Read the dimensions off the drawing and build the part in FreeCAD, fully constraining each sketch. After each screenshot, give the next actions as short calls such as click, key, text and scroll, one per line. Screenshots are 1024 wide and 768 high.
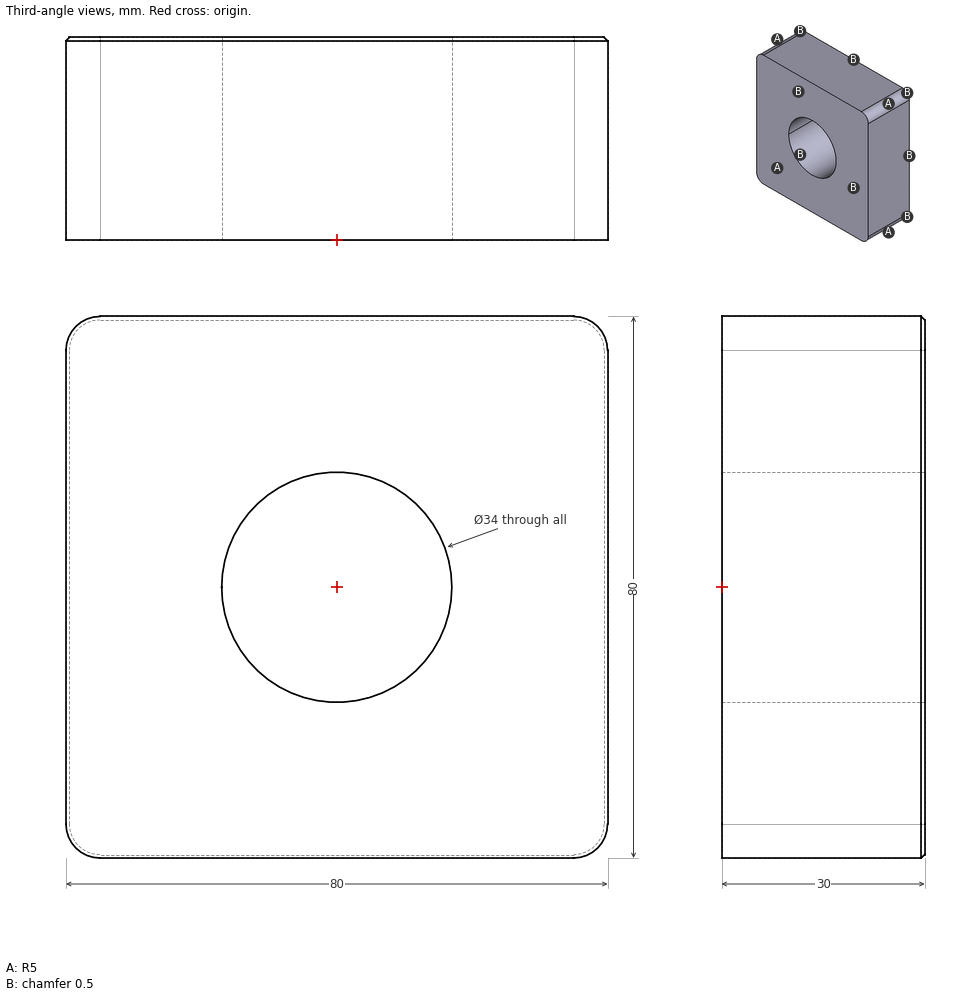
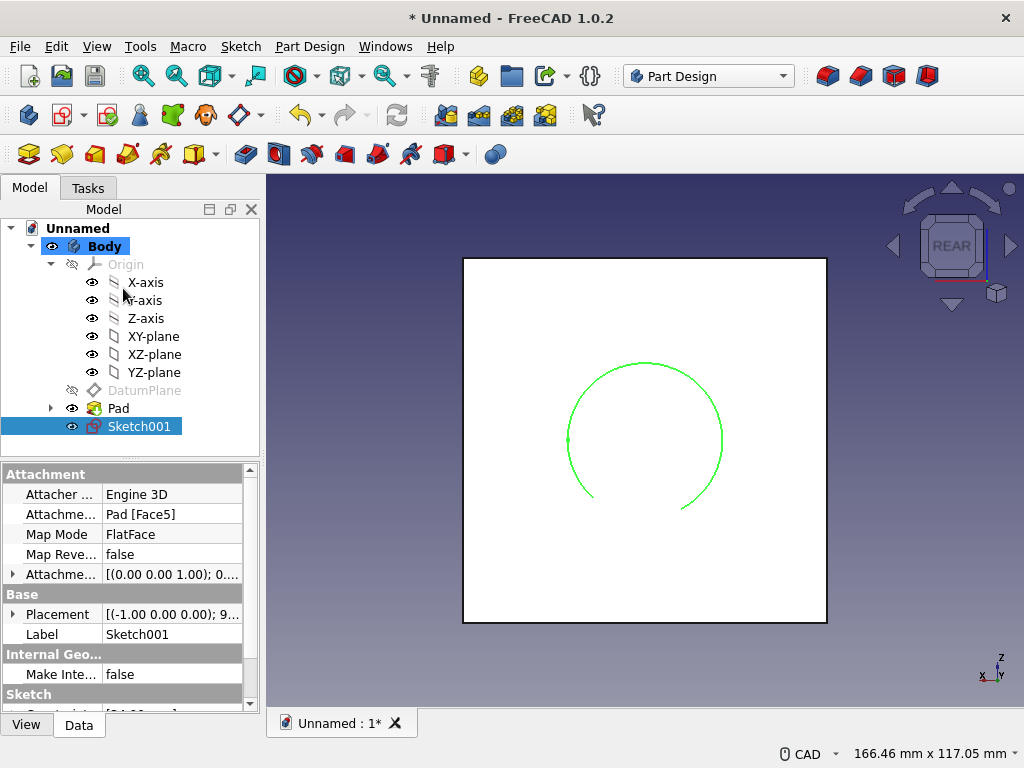
click(279, 154)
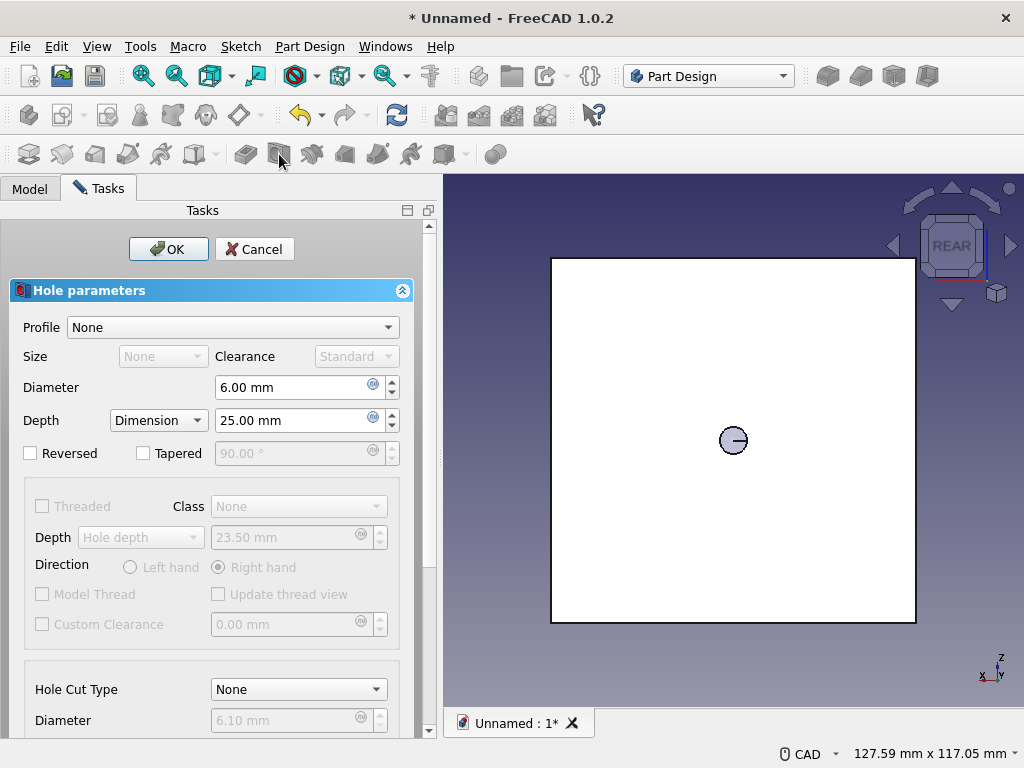
triple_click(300, 388)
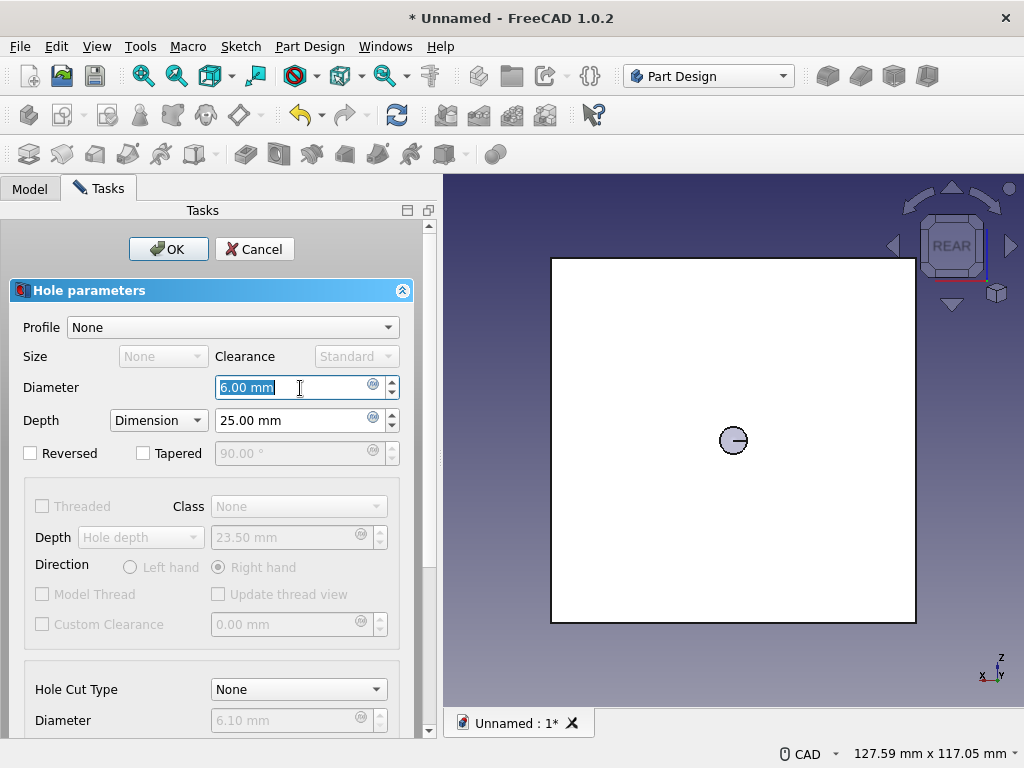
text(34)
key(Tab)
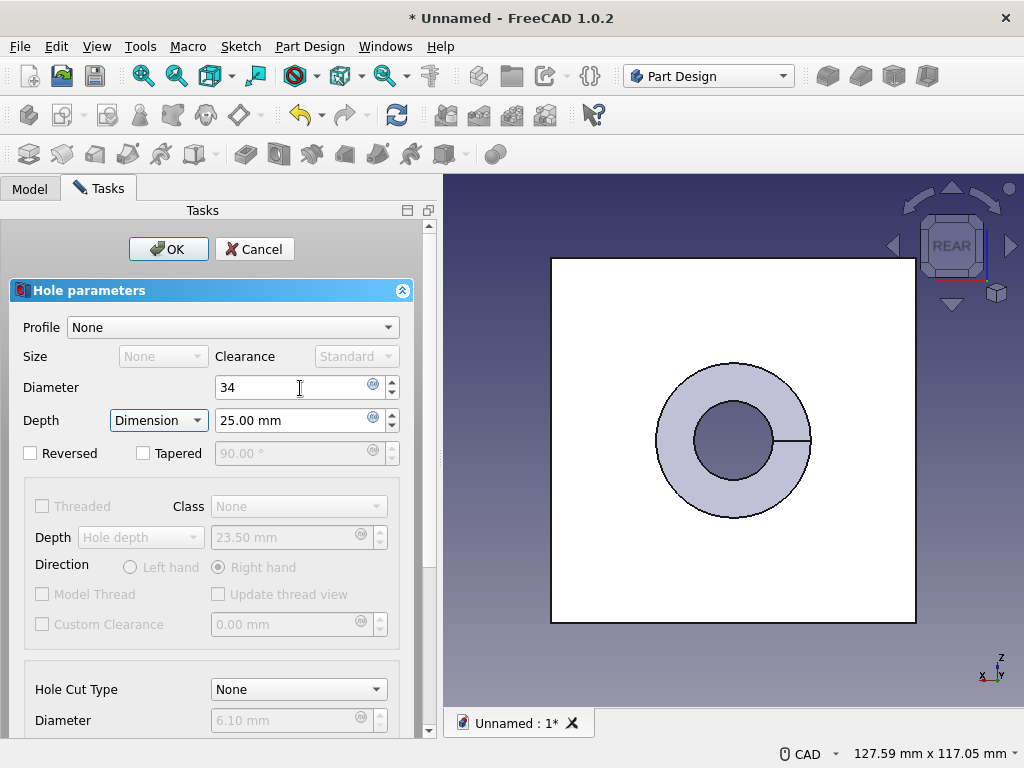
click(160, 420)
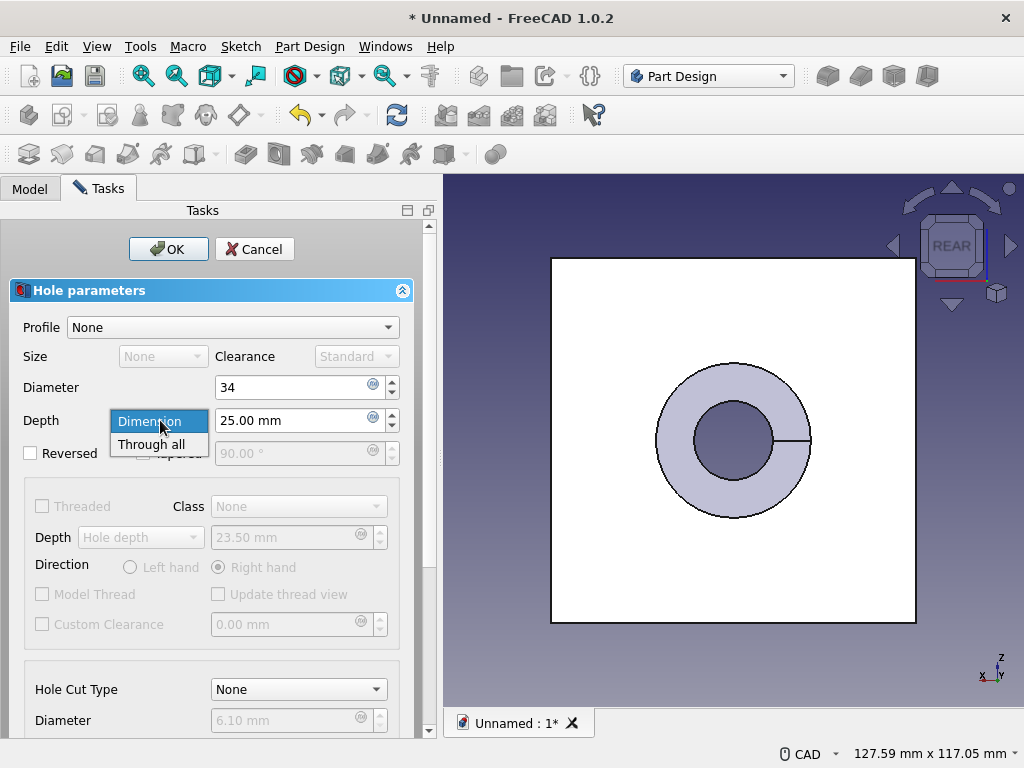
click(158, 444)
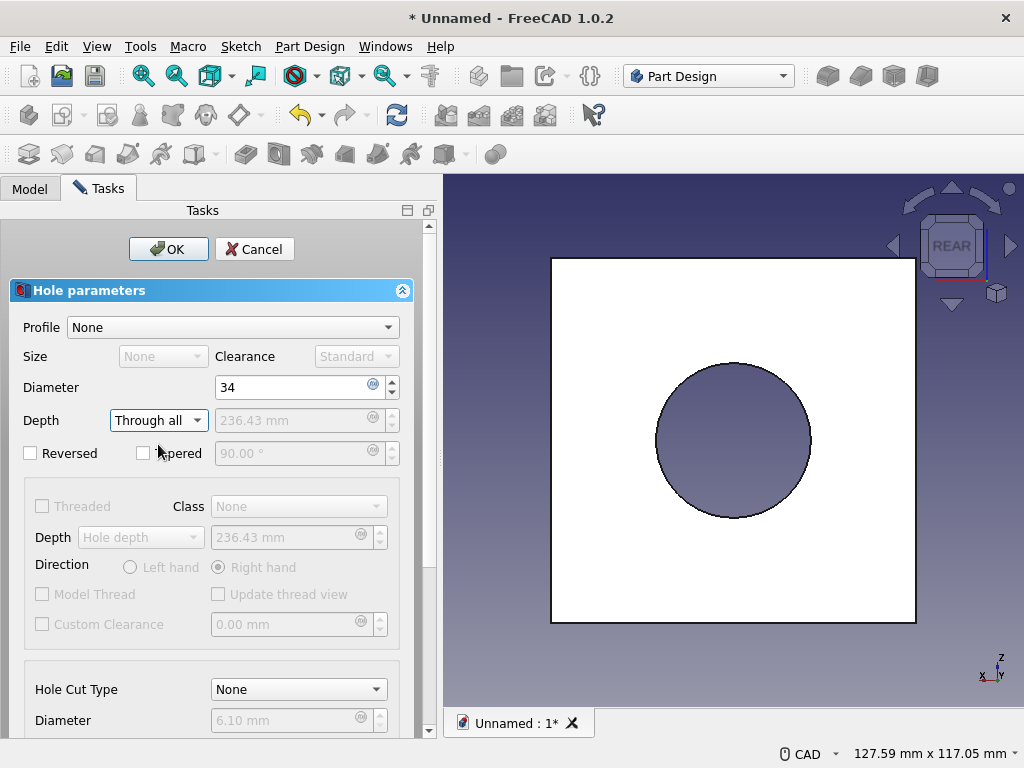
click(169, 249)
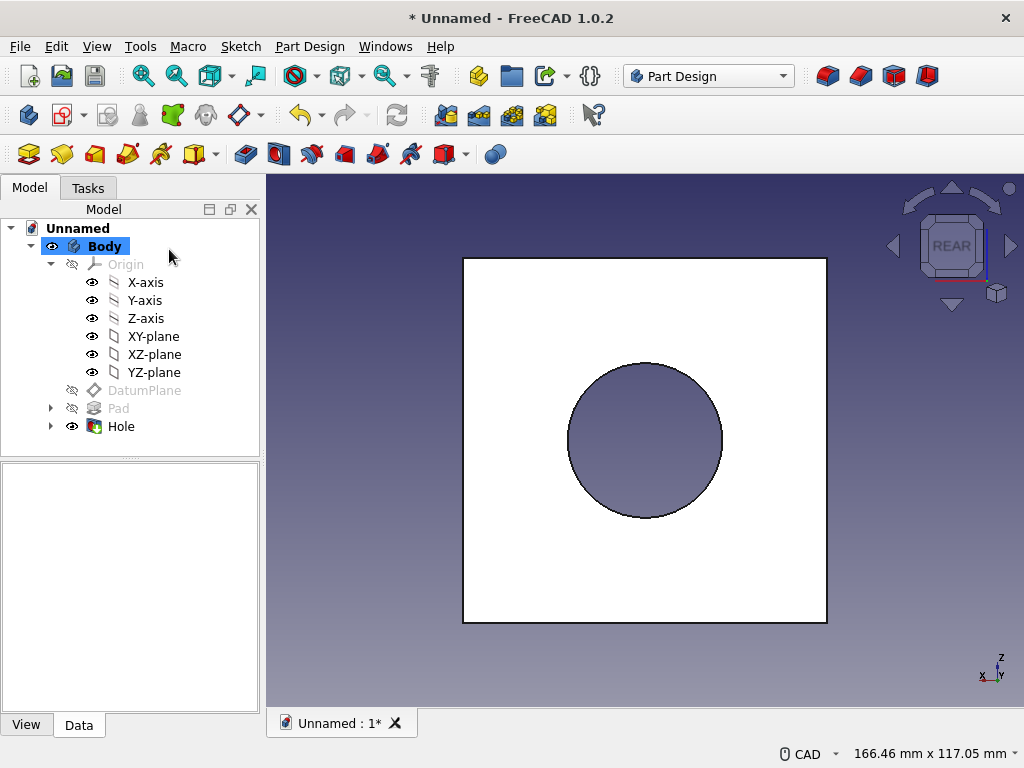
key(0)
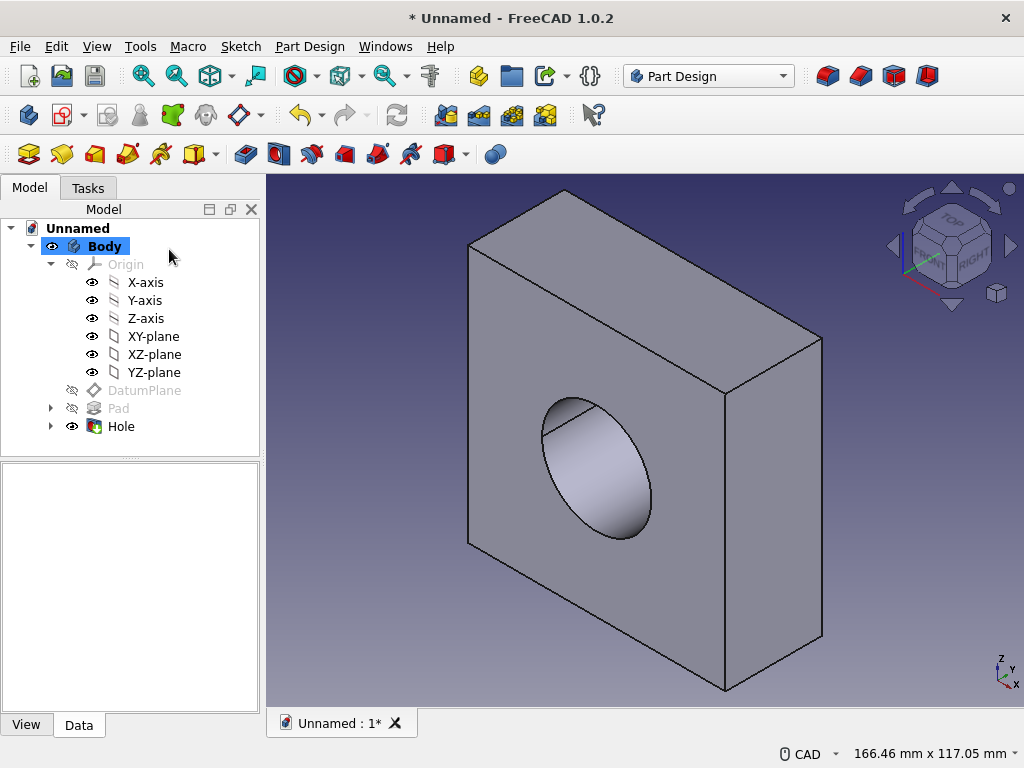
click(774, 365)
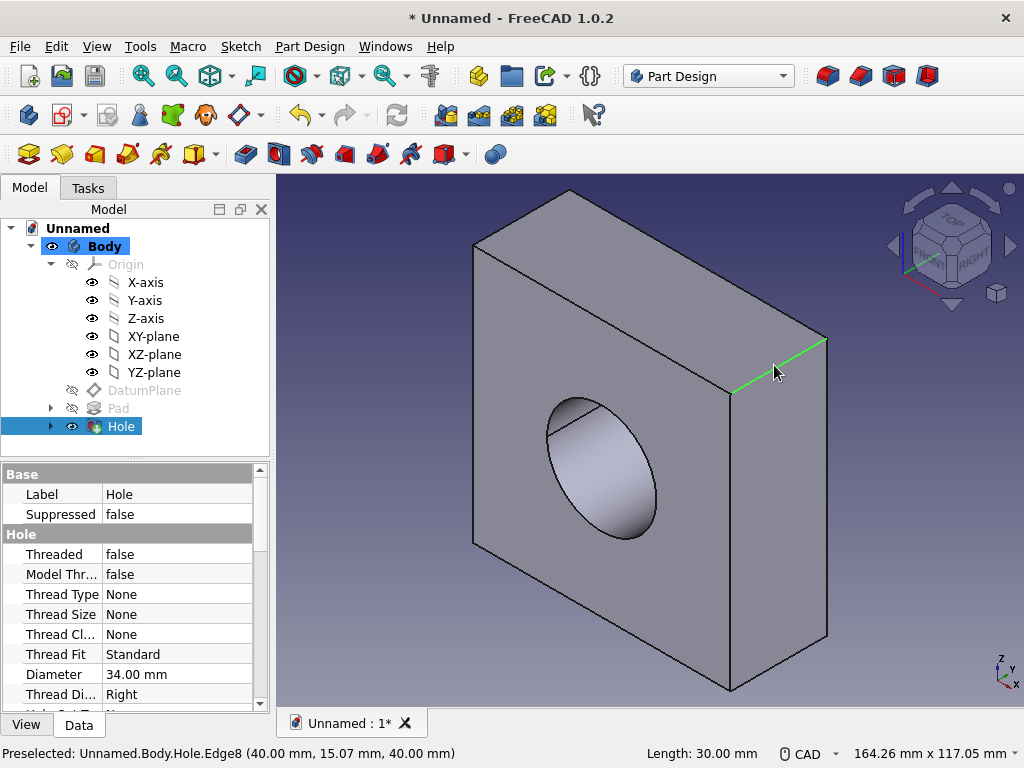
key(2)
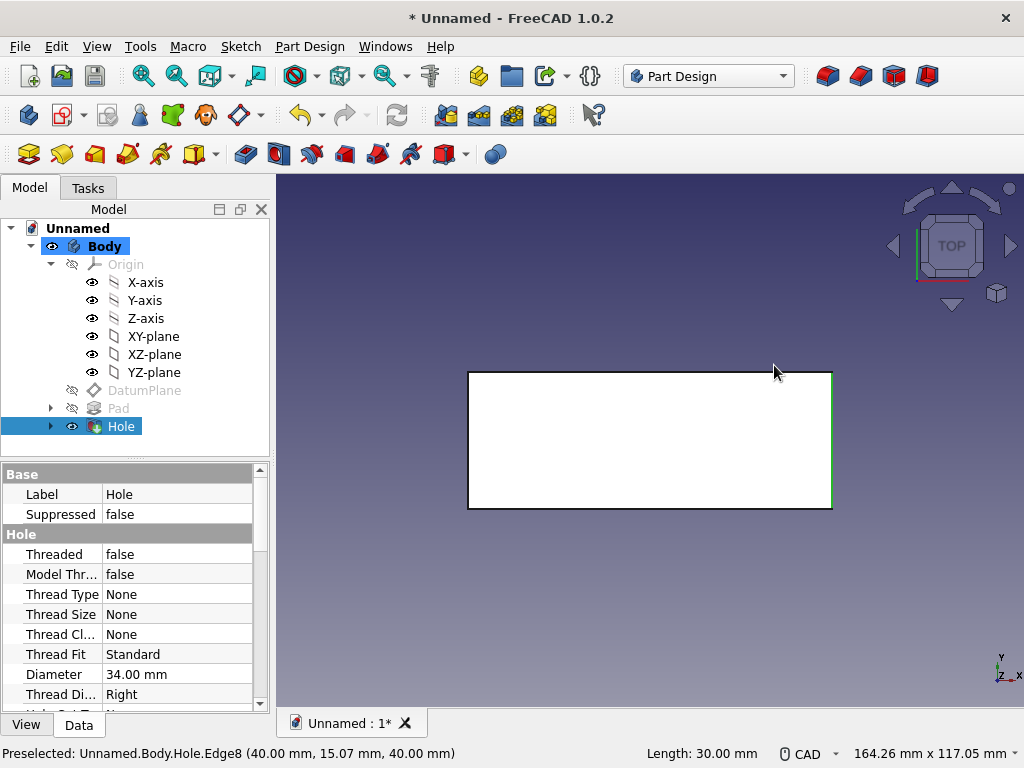
click(468, 439, ctrl)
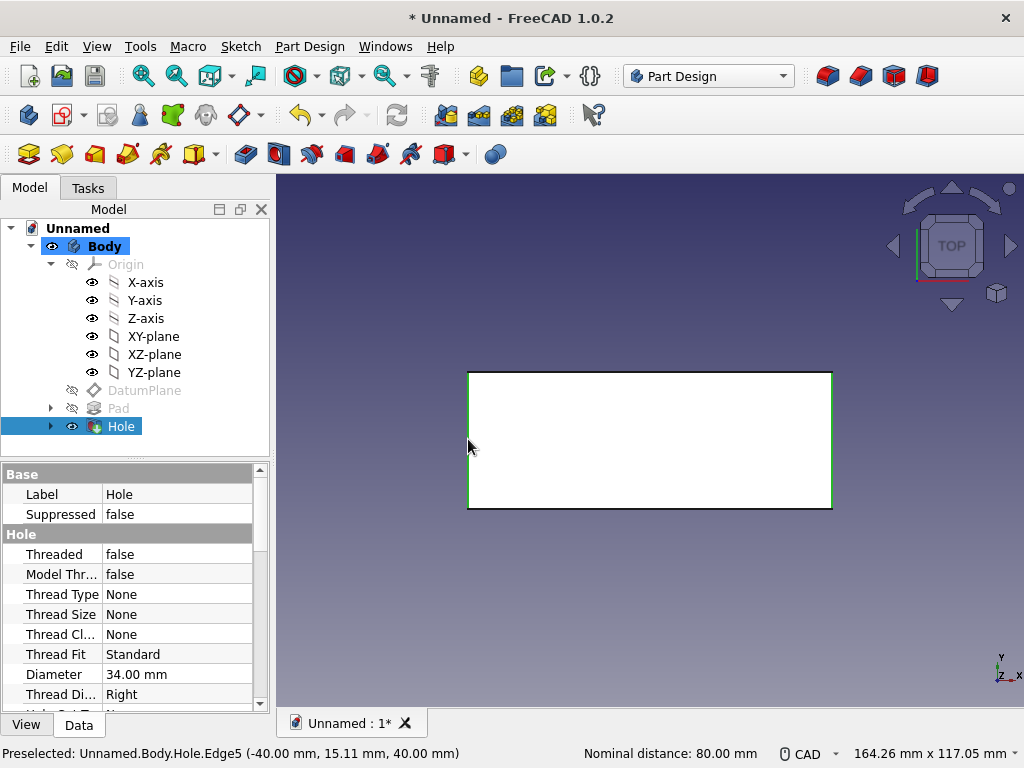
key(1)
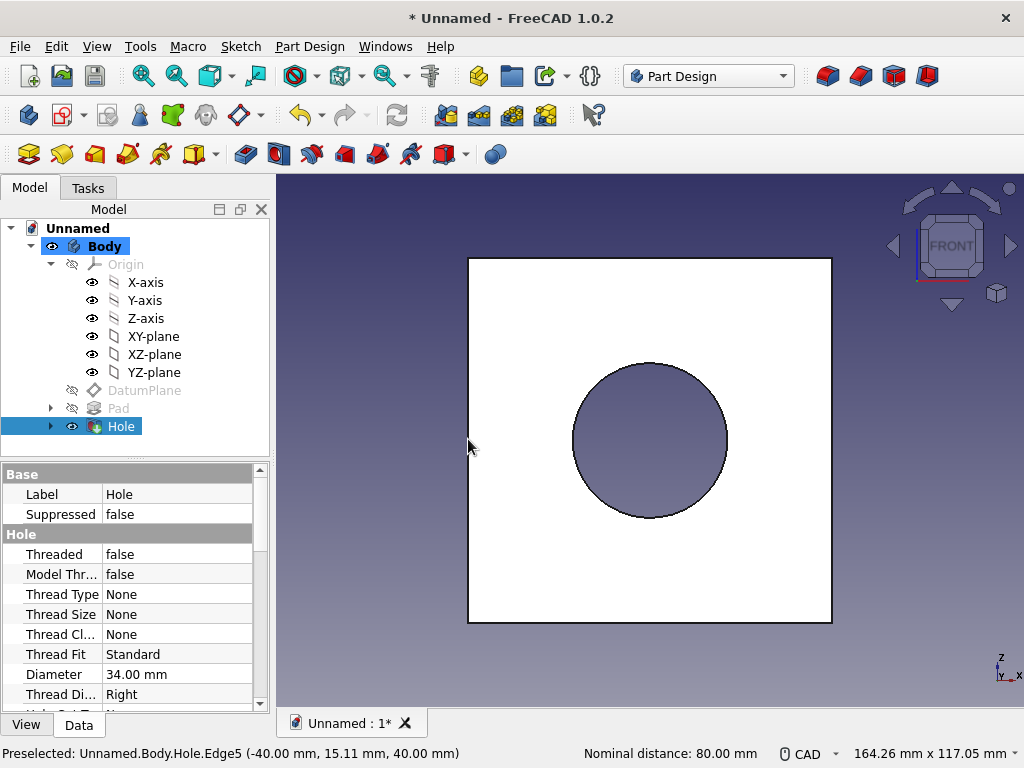
key(3)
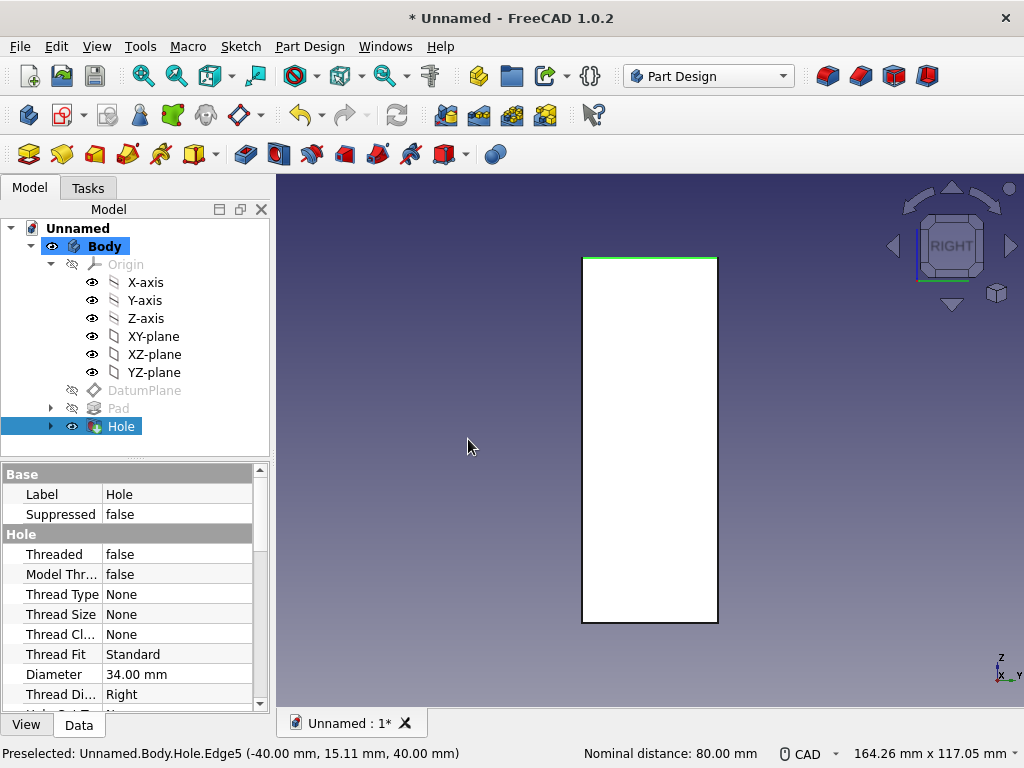
click(650, 622, ctrl)